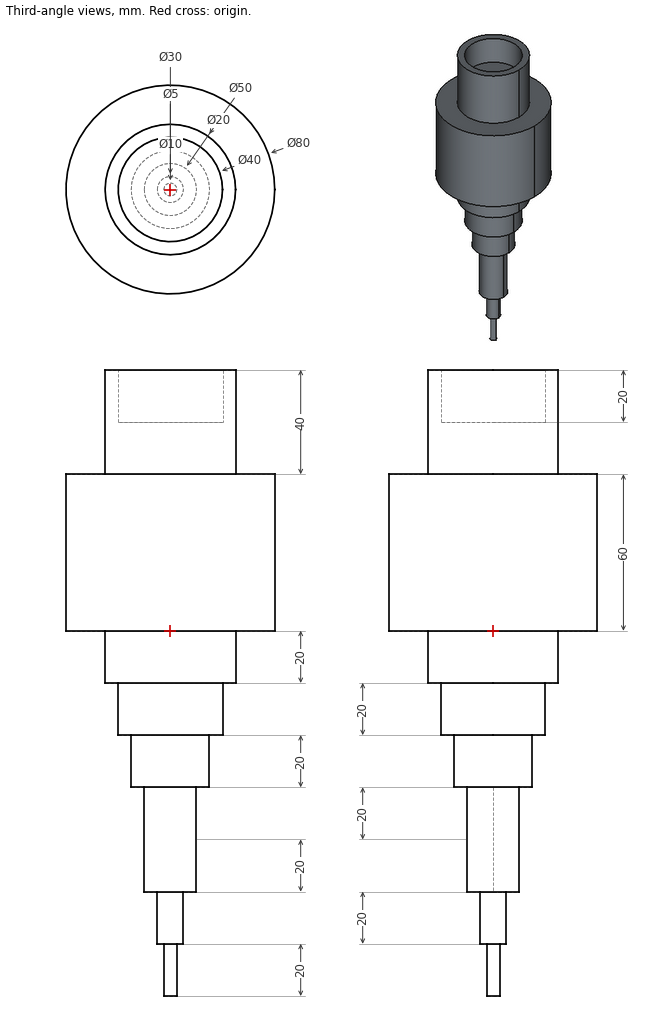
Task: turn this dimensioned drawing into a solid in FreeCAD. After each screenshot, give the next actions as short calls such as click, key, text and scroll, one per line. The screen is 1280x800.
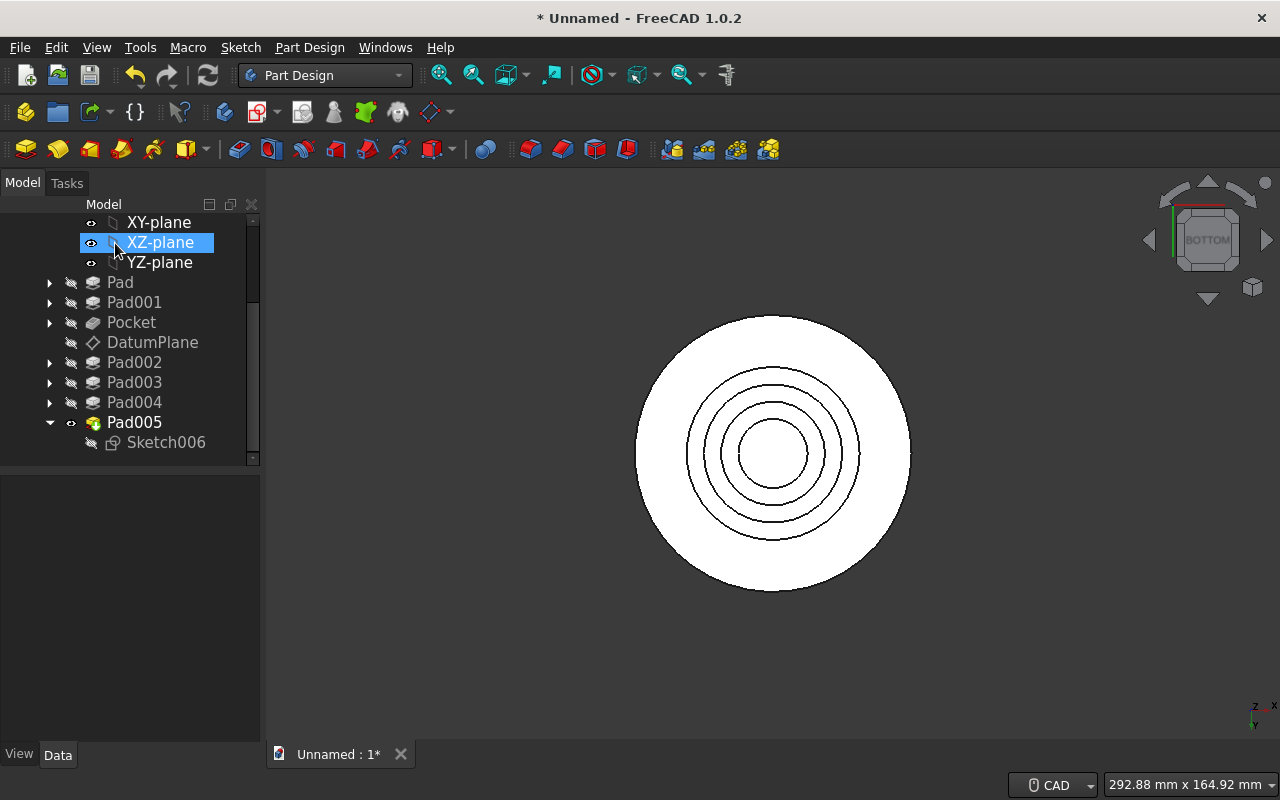
click(773, 452)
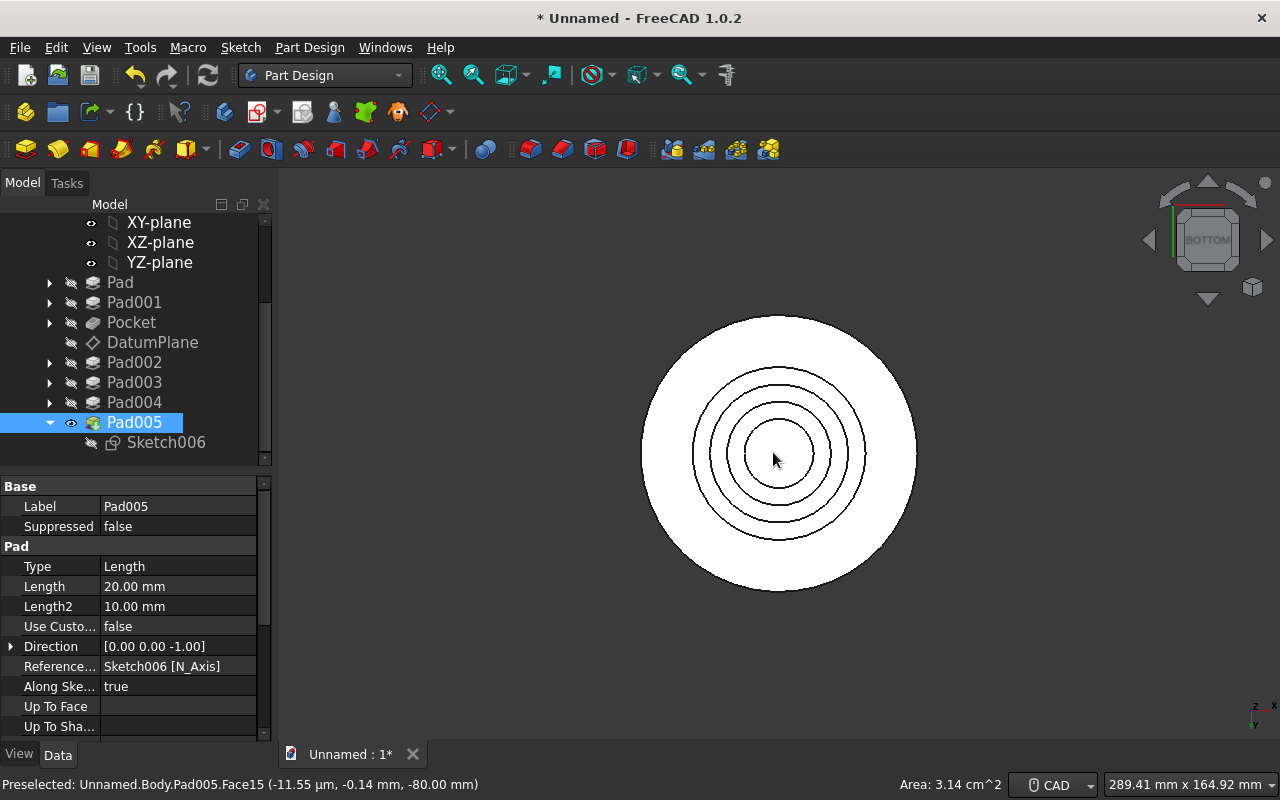
click(258, 112)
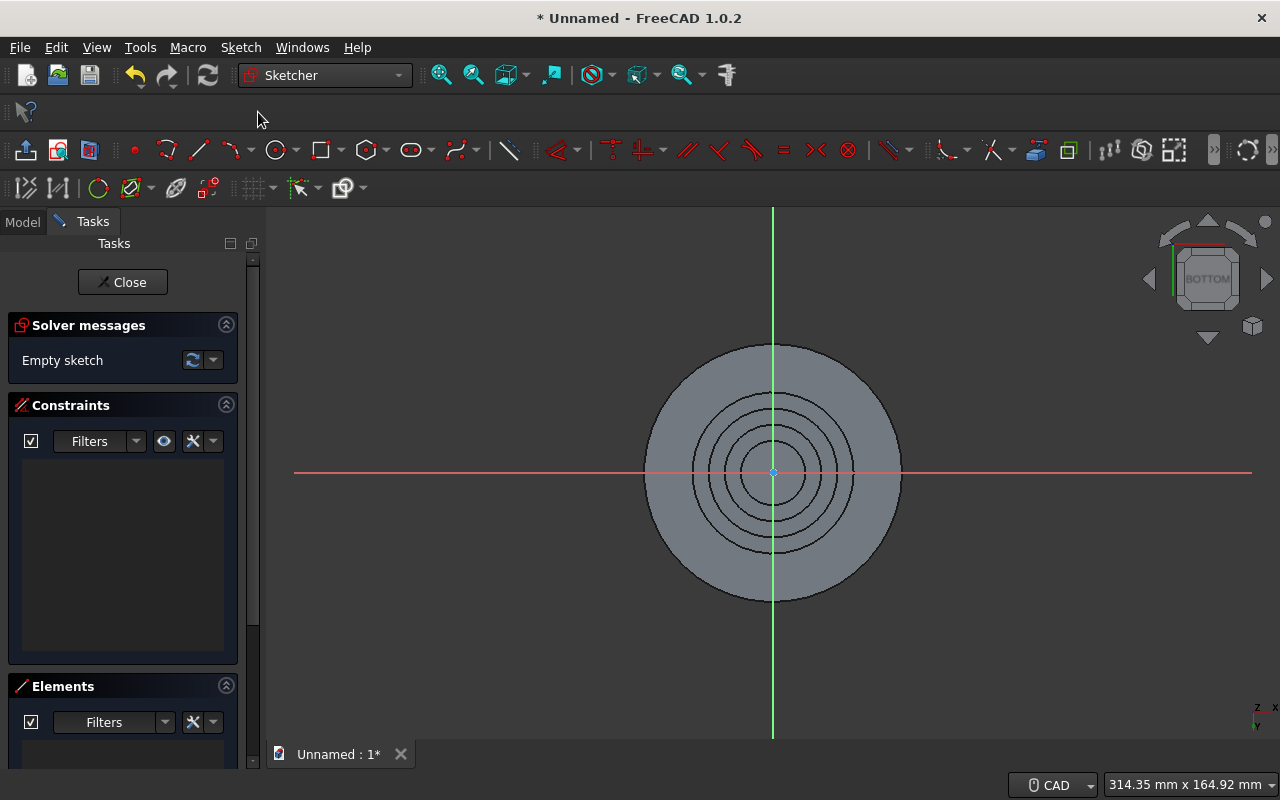
scroll(790, 473, up, 8)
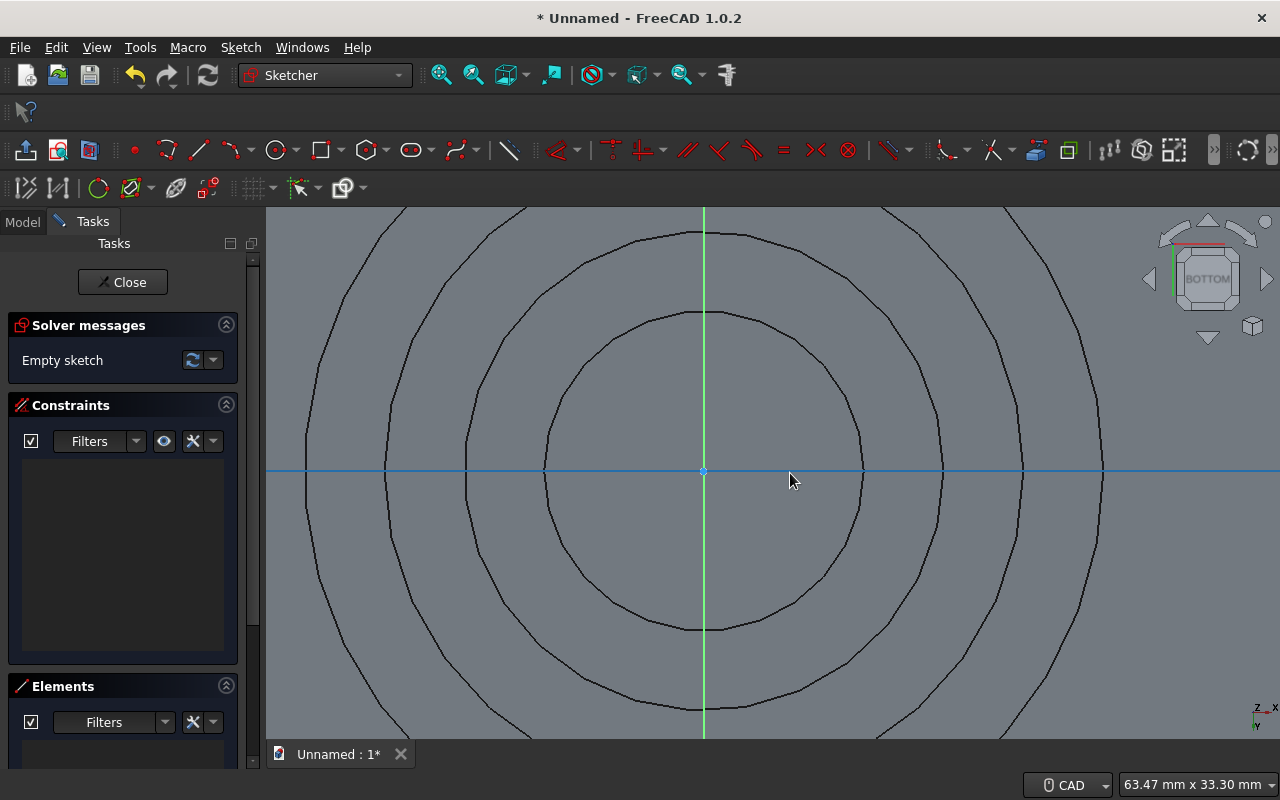
click(276, 150)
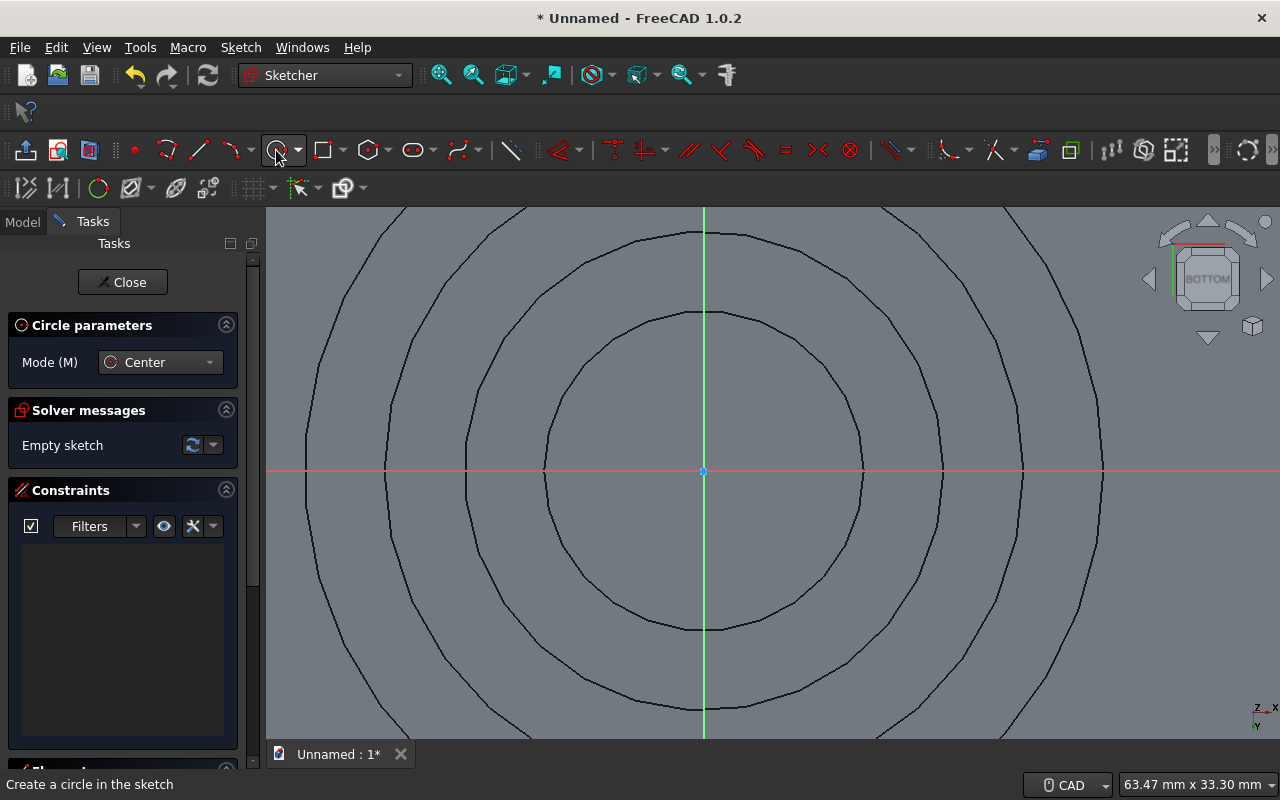
click(704, 471)
click(817, 358)
key(Escape)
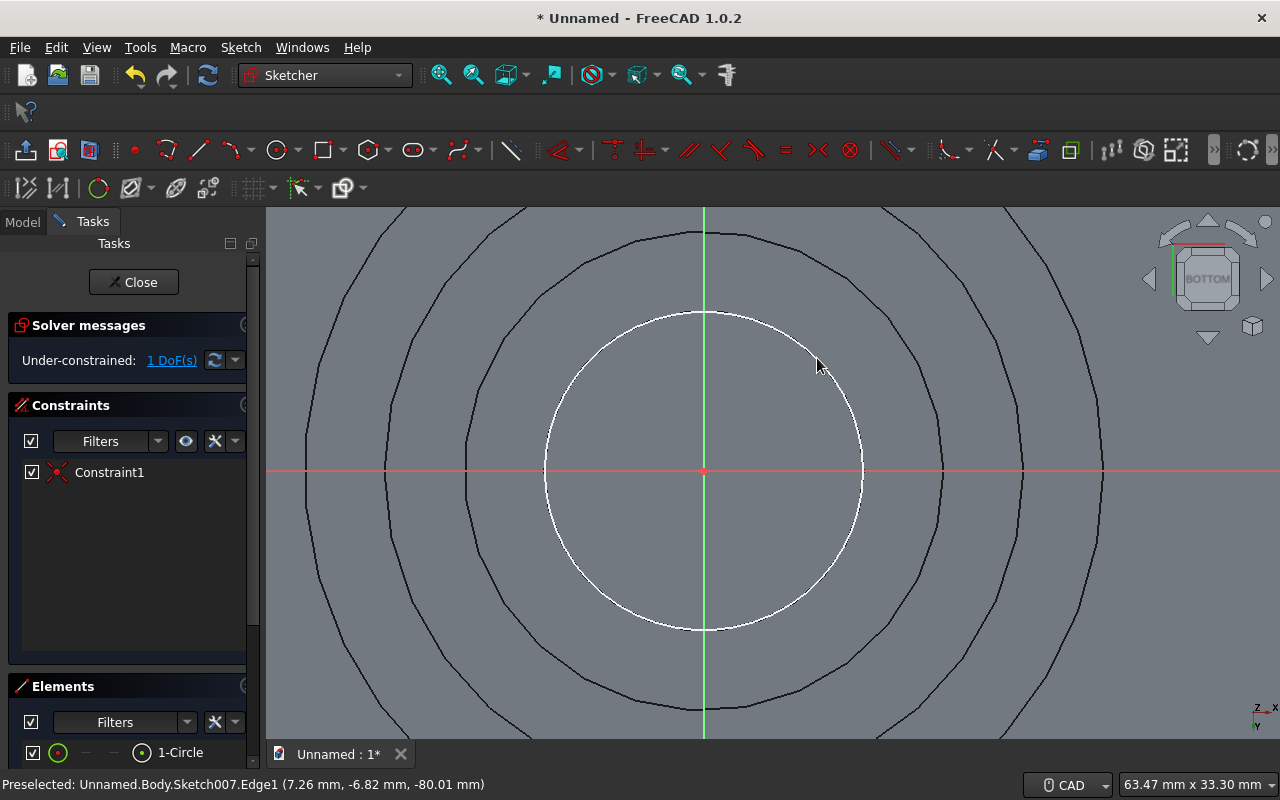
click(558, 150)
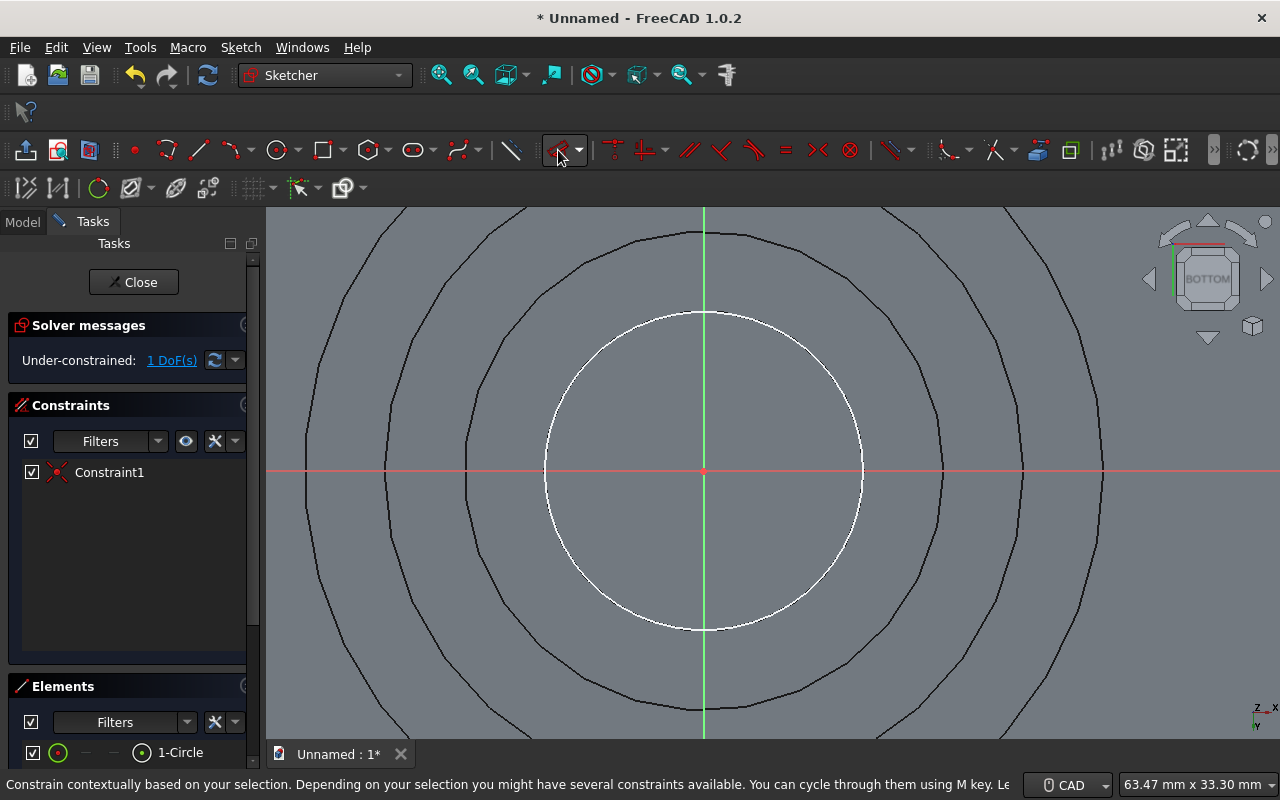
click(816, 358)
click(839, 335)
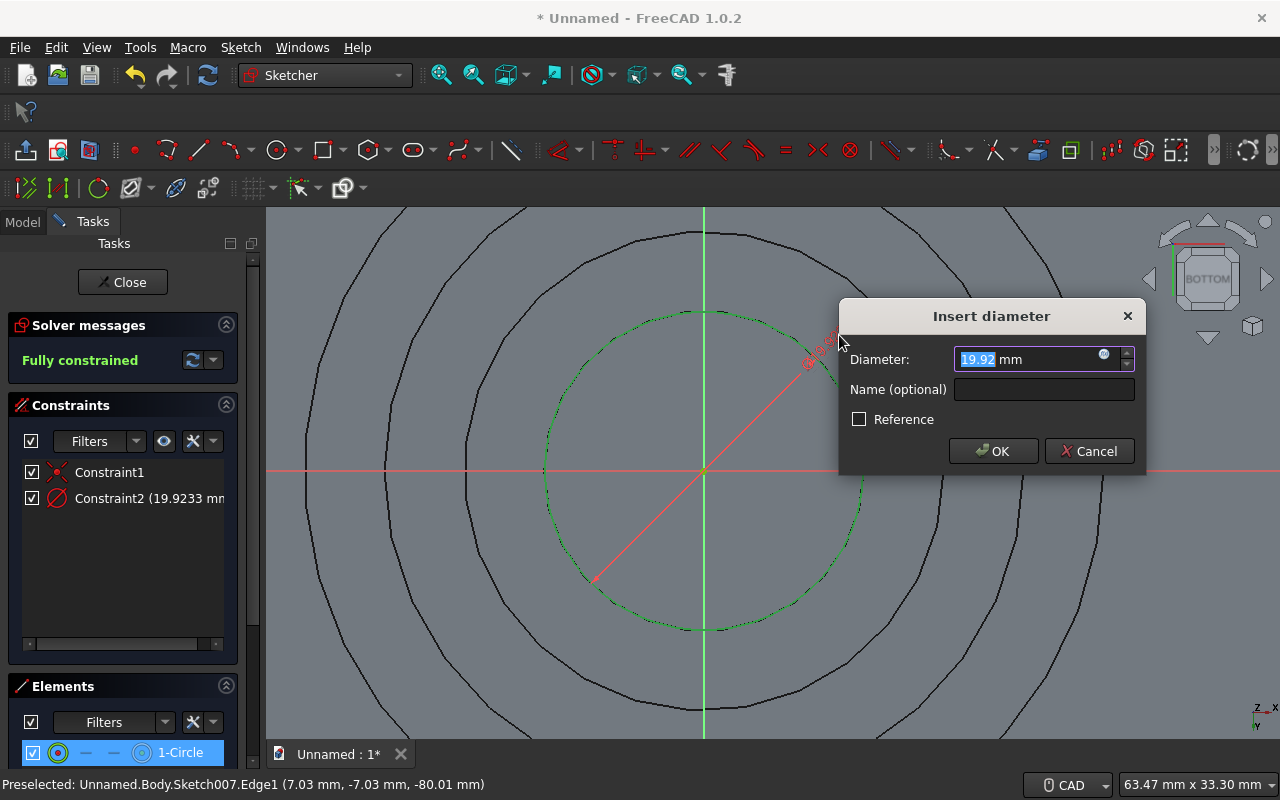
text(20)
key(Return)
key(Escape)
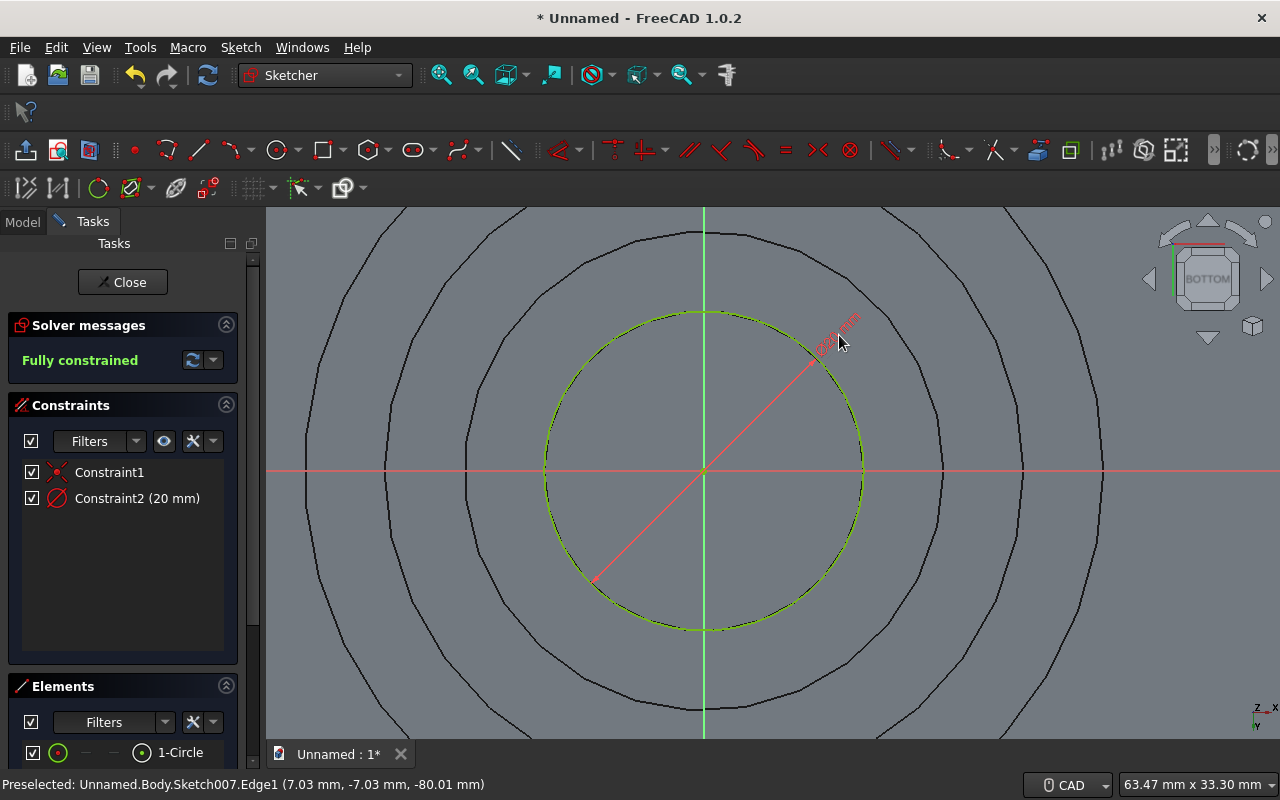
click(123, 282)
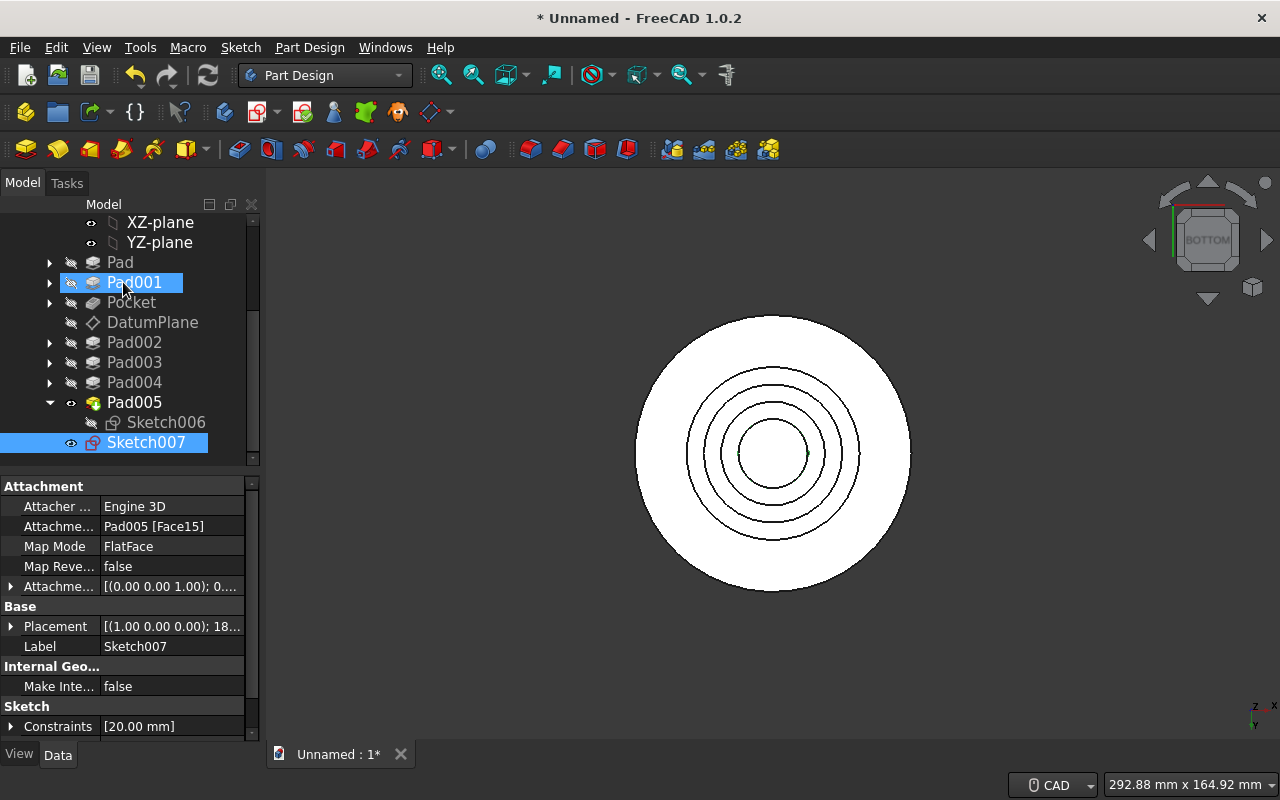
click(26, 150)